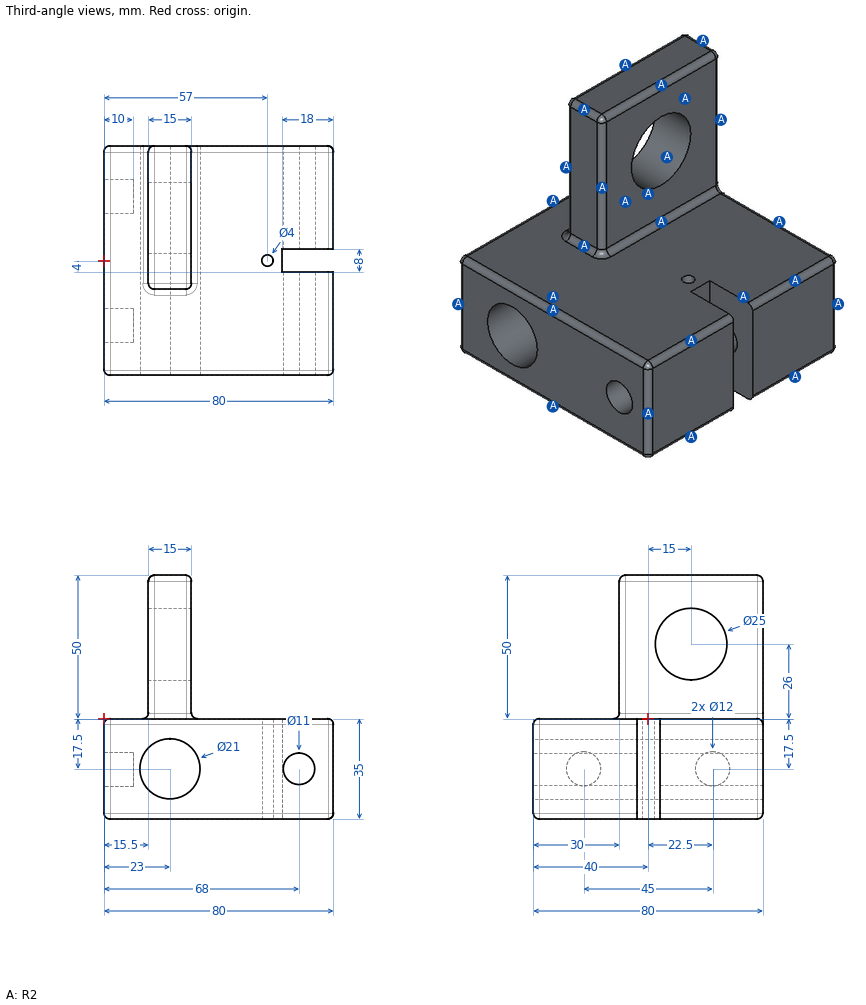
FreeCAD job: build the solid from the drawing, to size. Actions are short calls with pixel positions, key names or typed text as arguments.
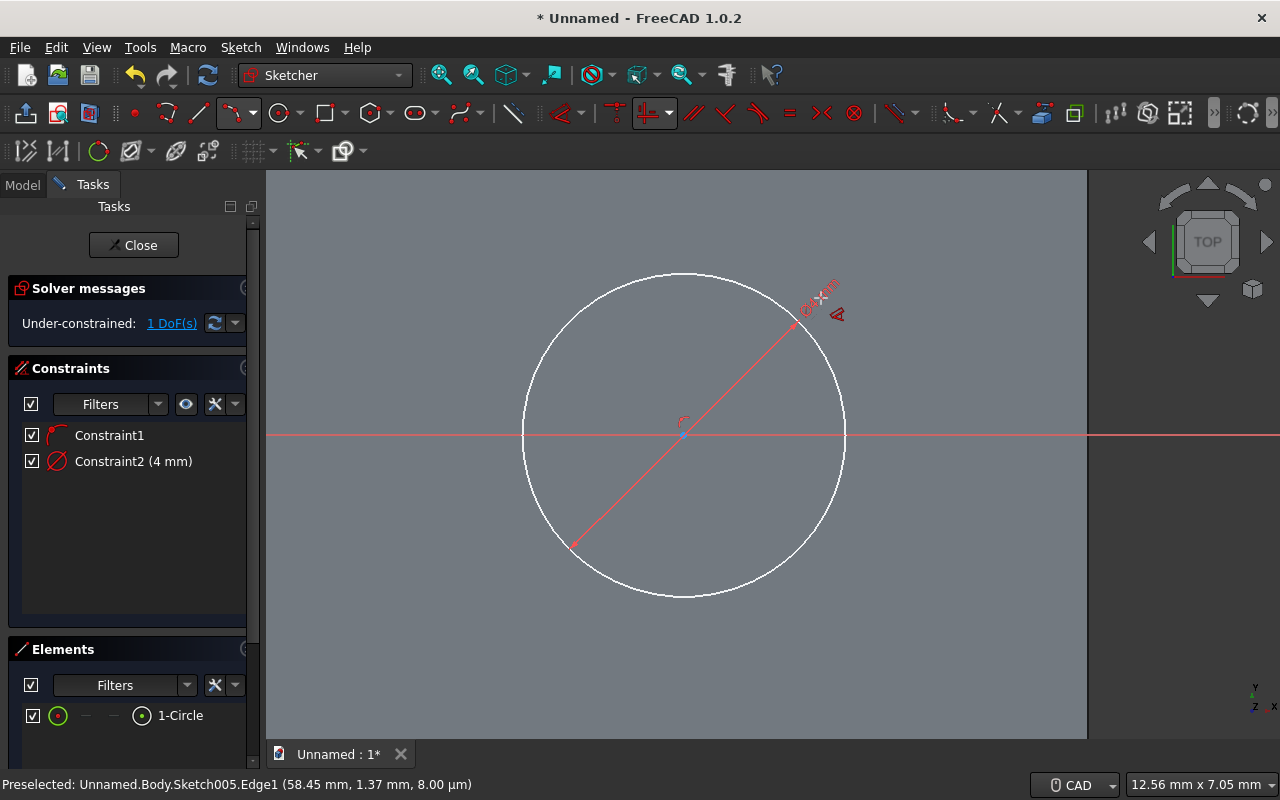
click(684, 435)
click(489, 469)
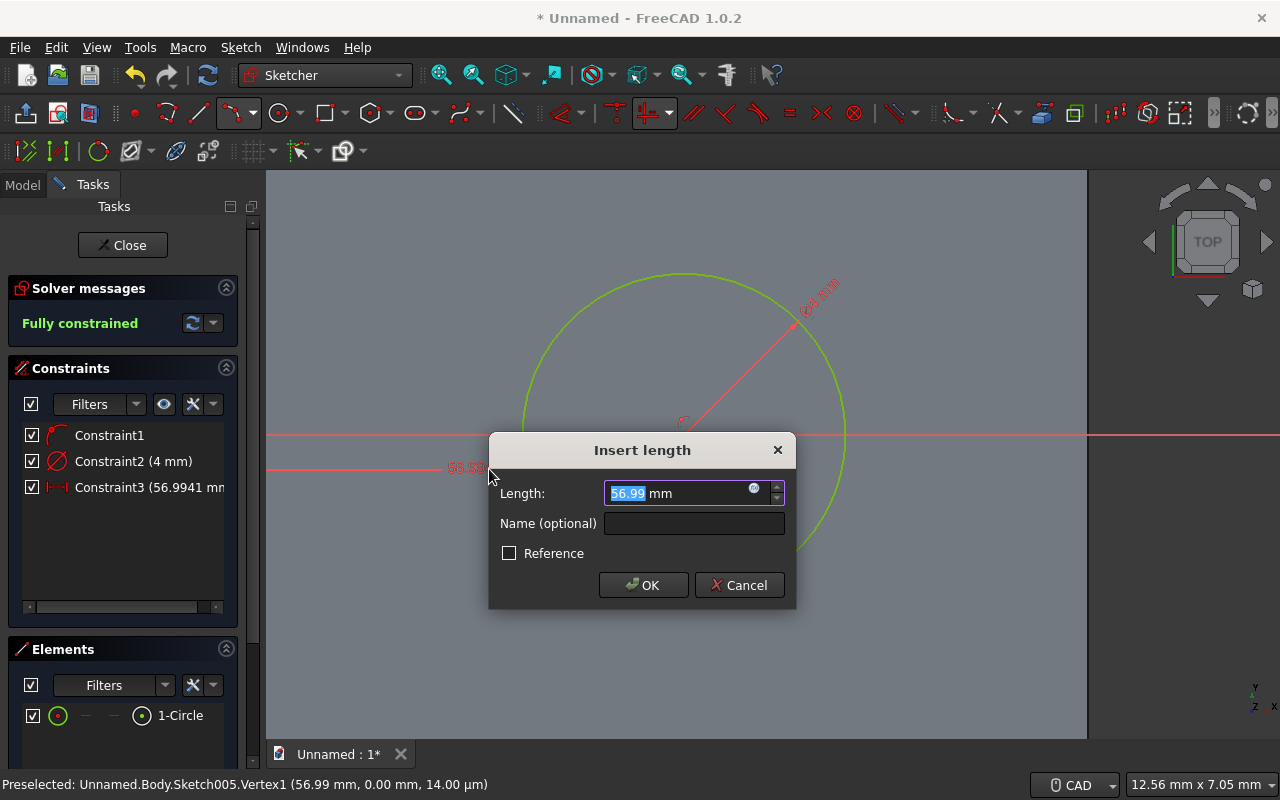
text(57)
key(Return)
key(Escape)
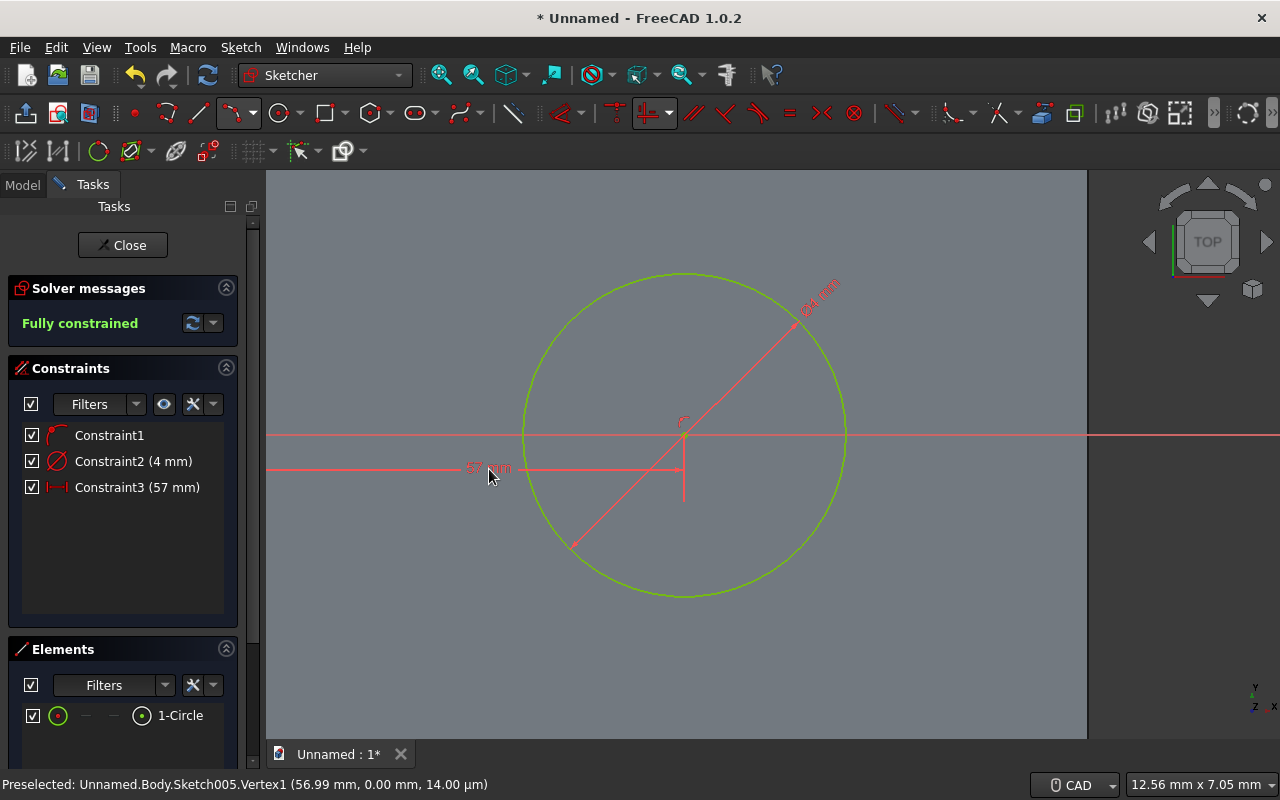
click(123, 245)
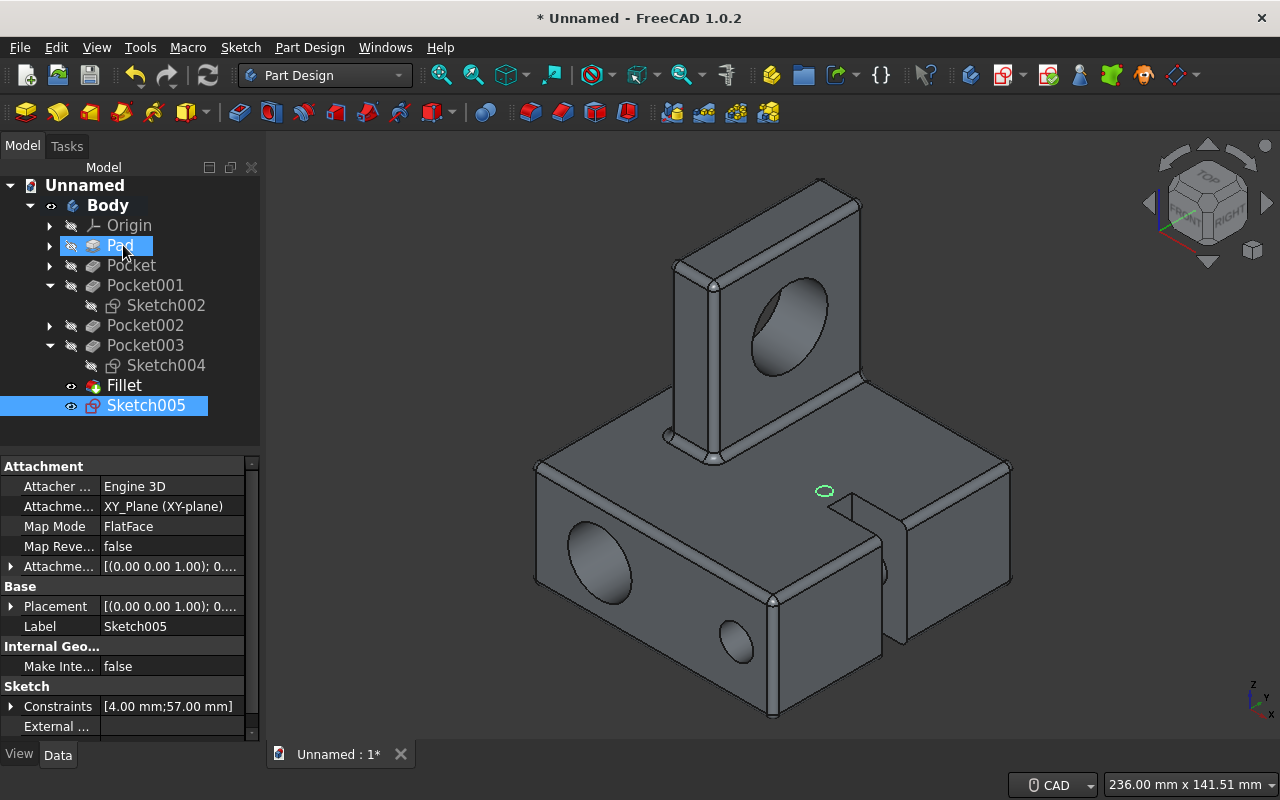
click(240, 112)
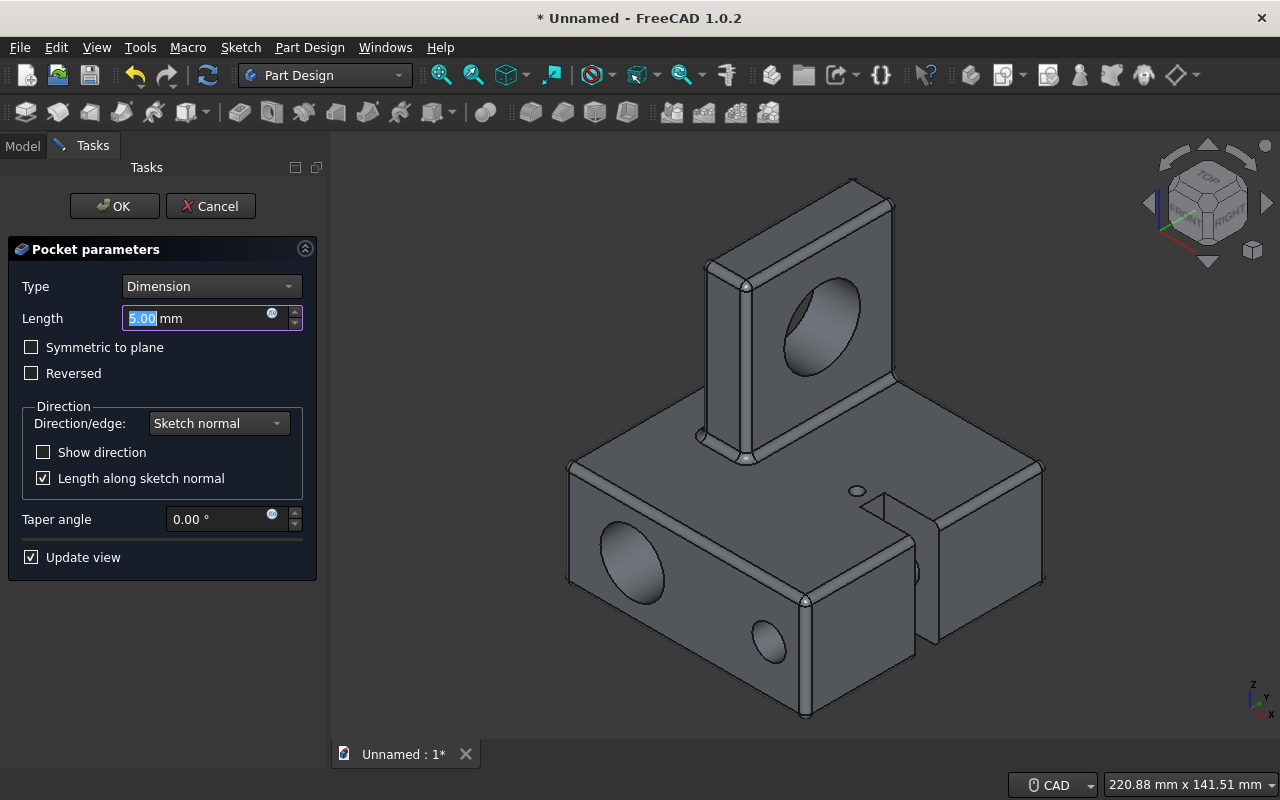
click(212, 286)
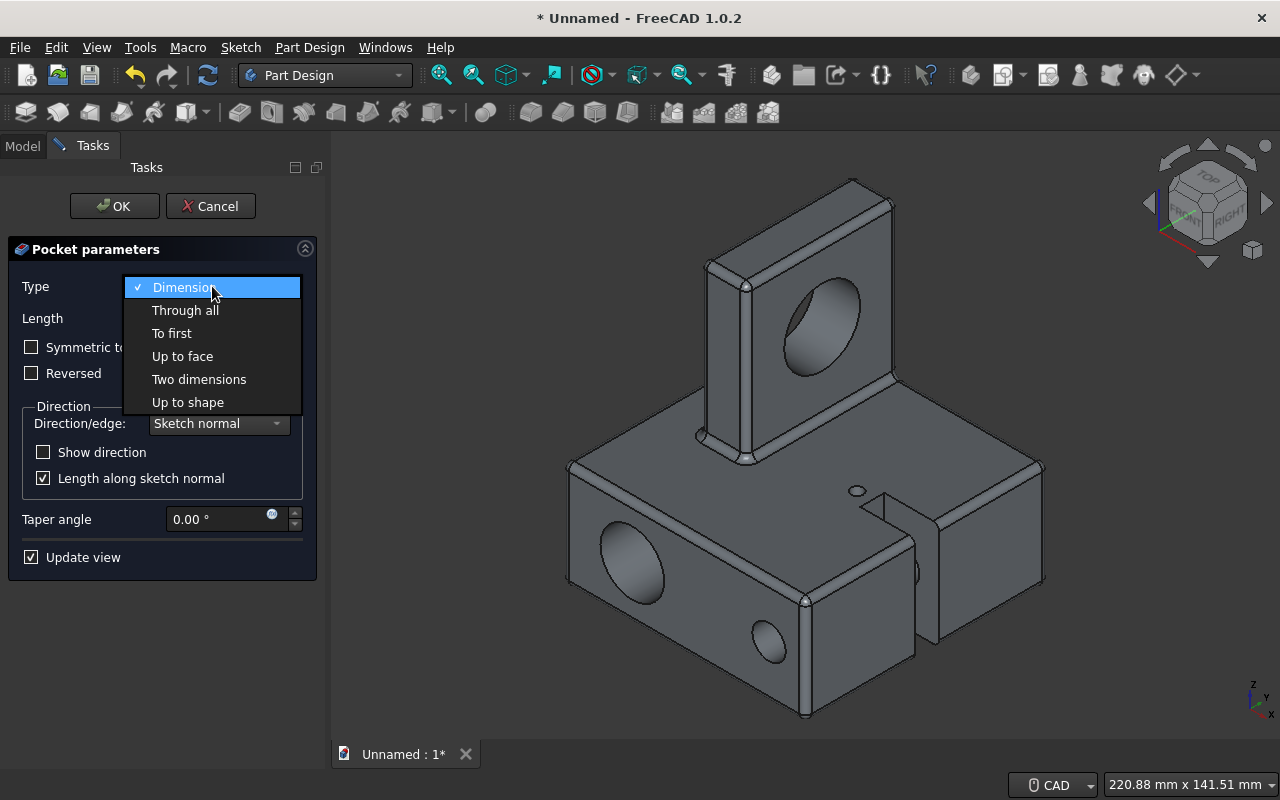
click(212, 310)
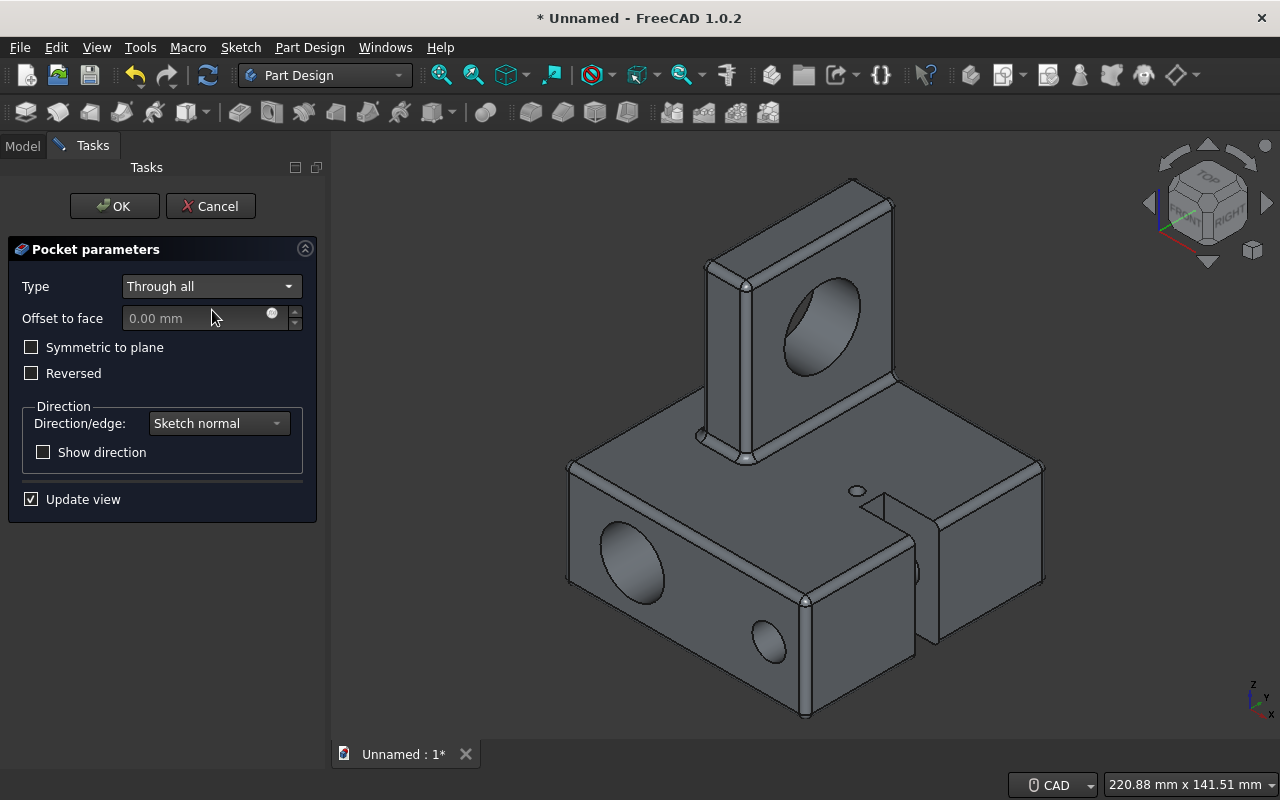
click(115, 206)